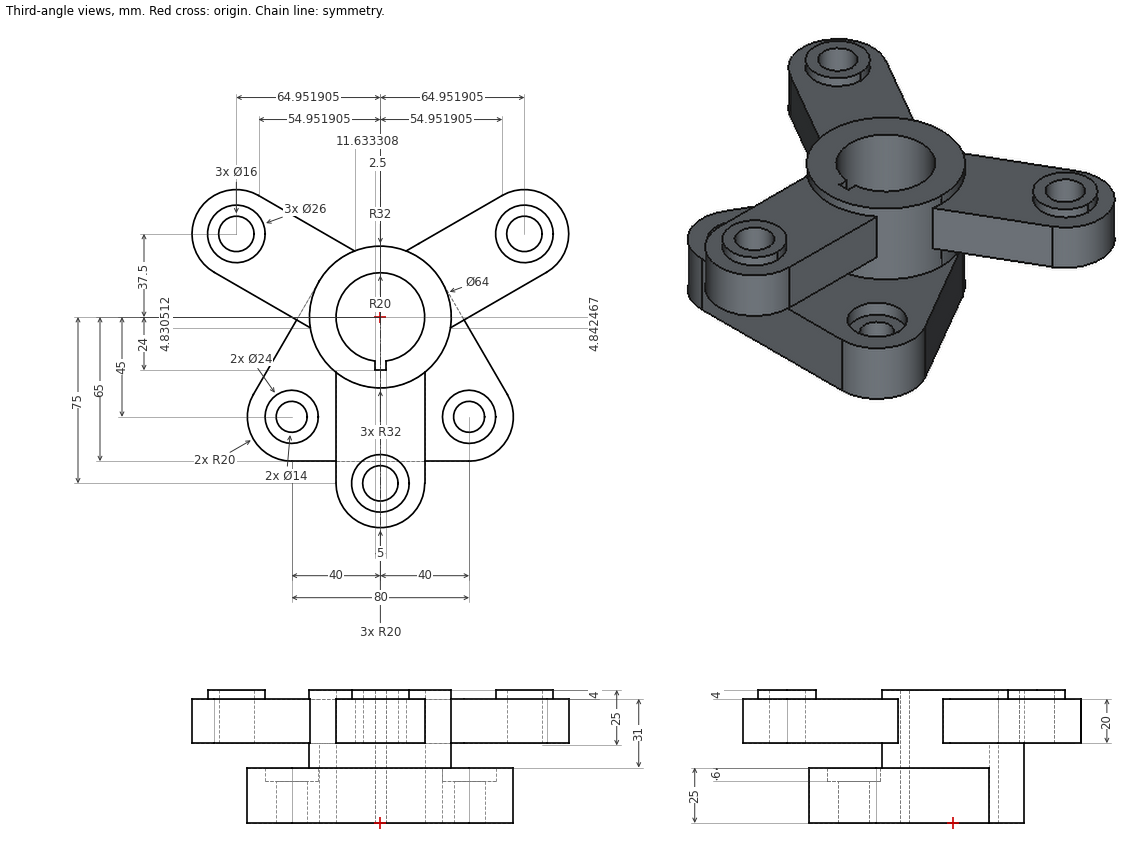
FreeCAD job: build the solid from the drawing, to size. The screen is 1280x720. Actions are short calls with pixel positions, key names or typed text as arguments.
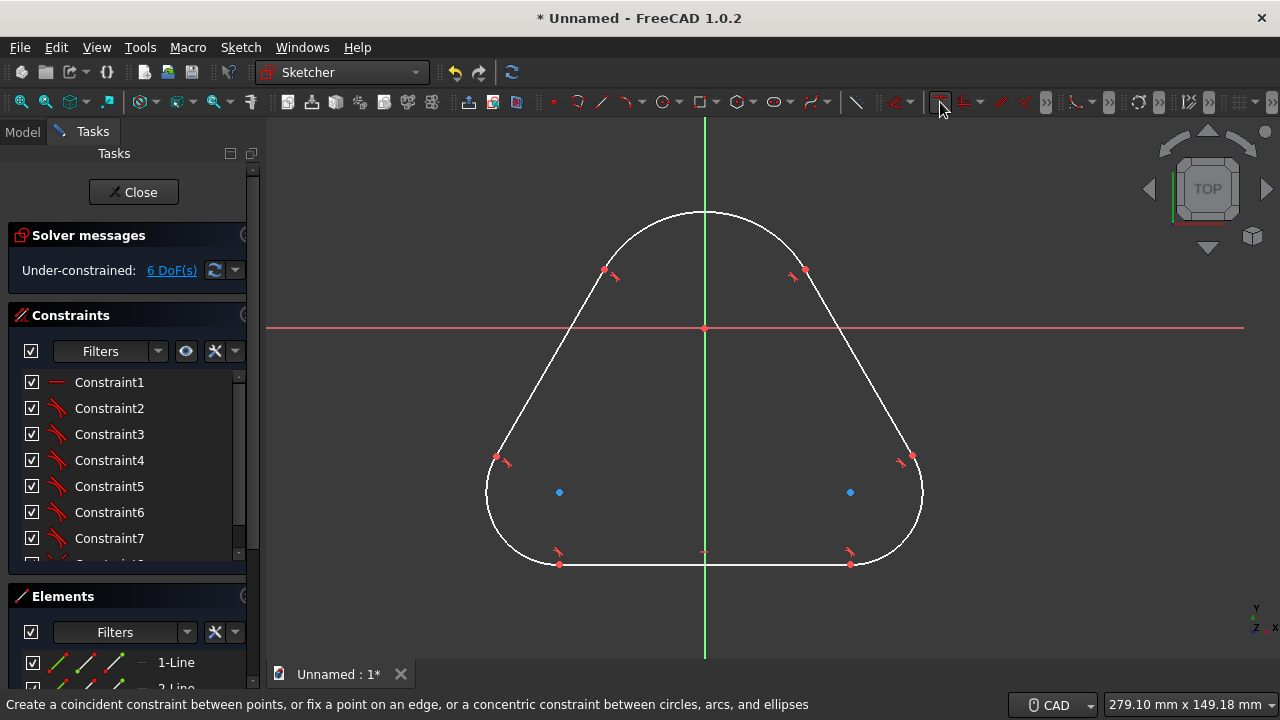
click(487, 500)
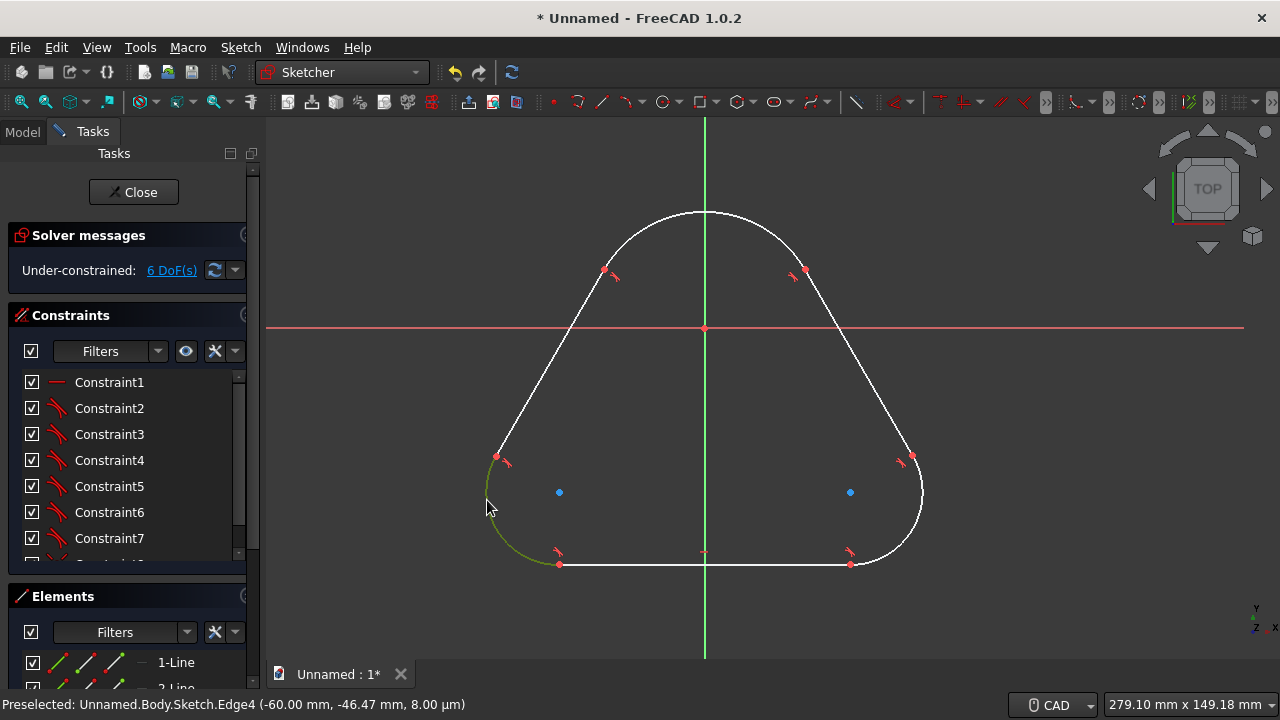
click(893, 551)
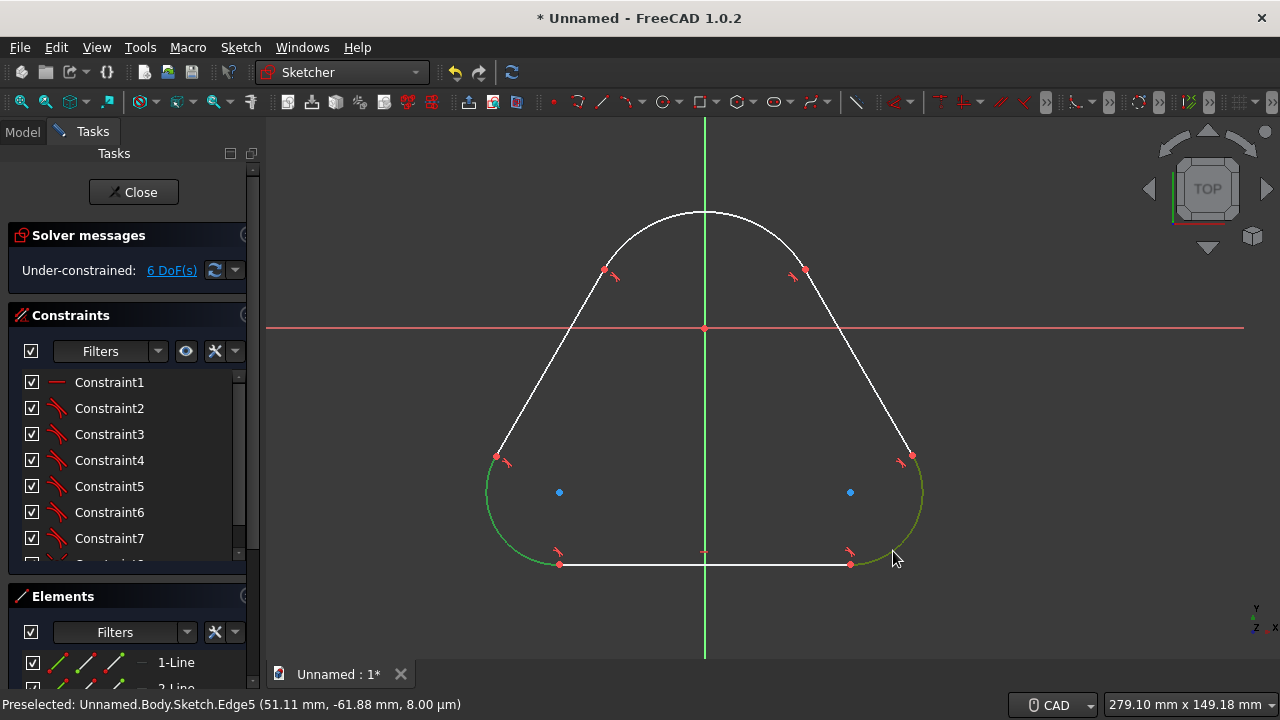
key(e)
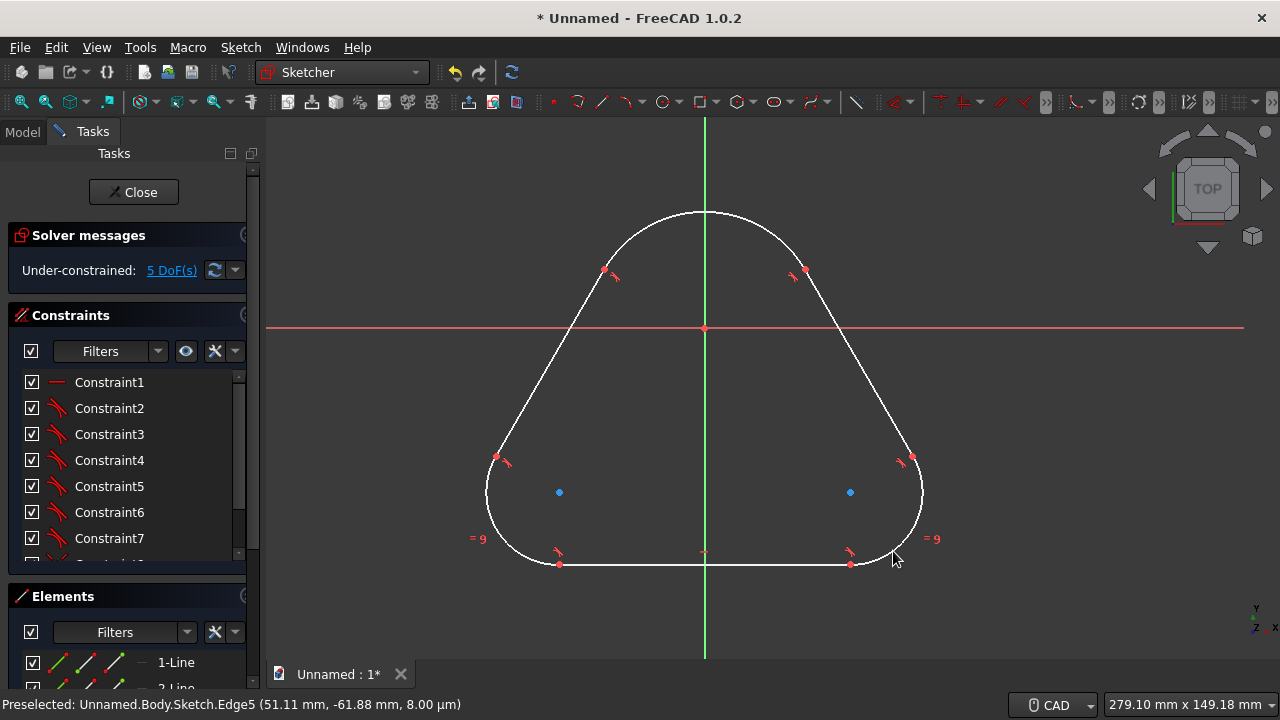
click(487, 500)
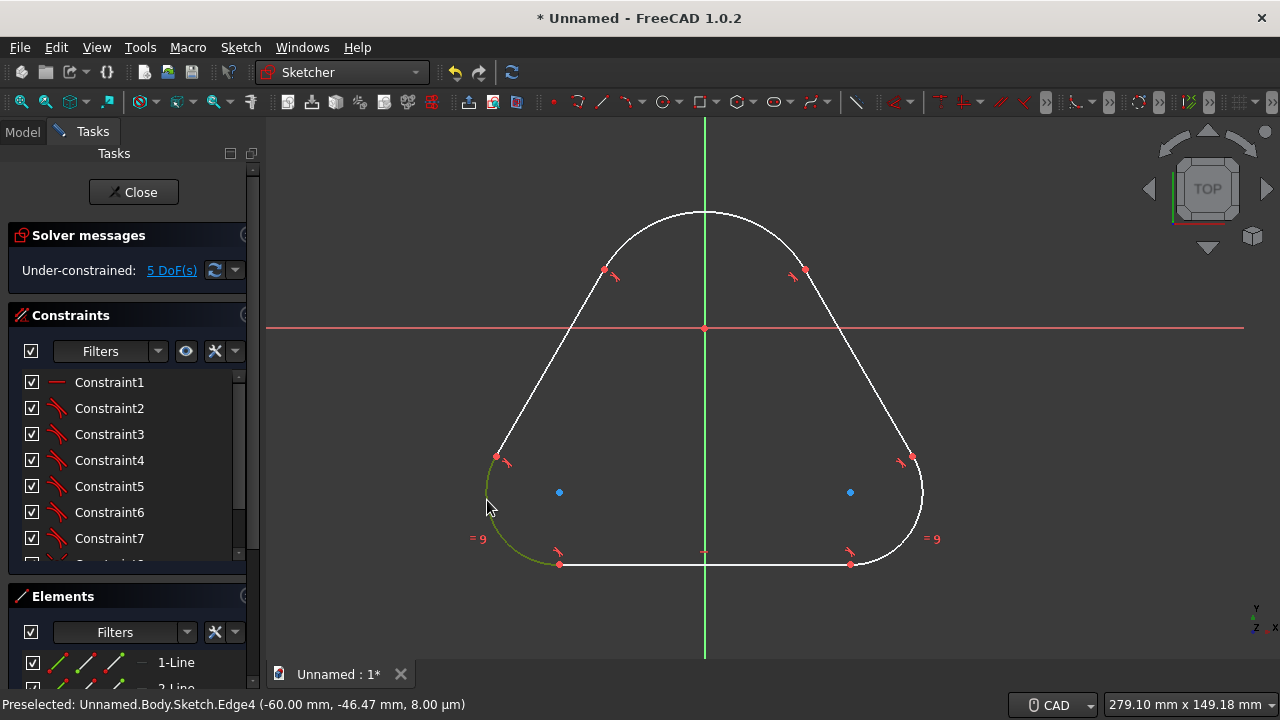
key(k)
key(r)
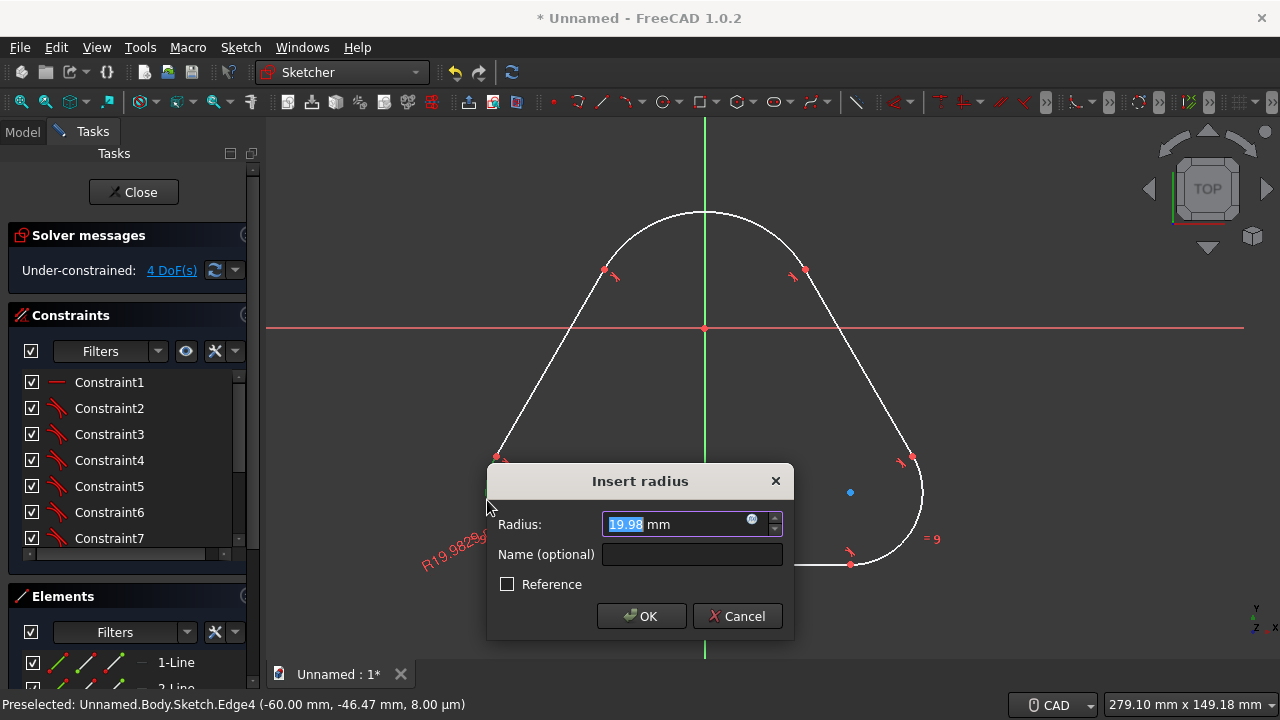
text(20)
key(Return)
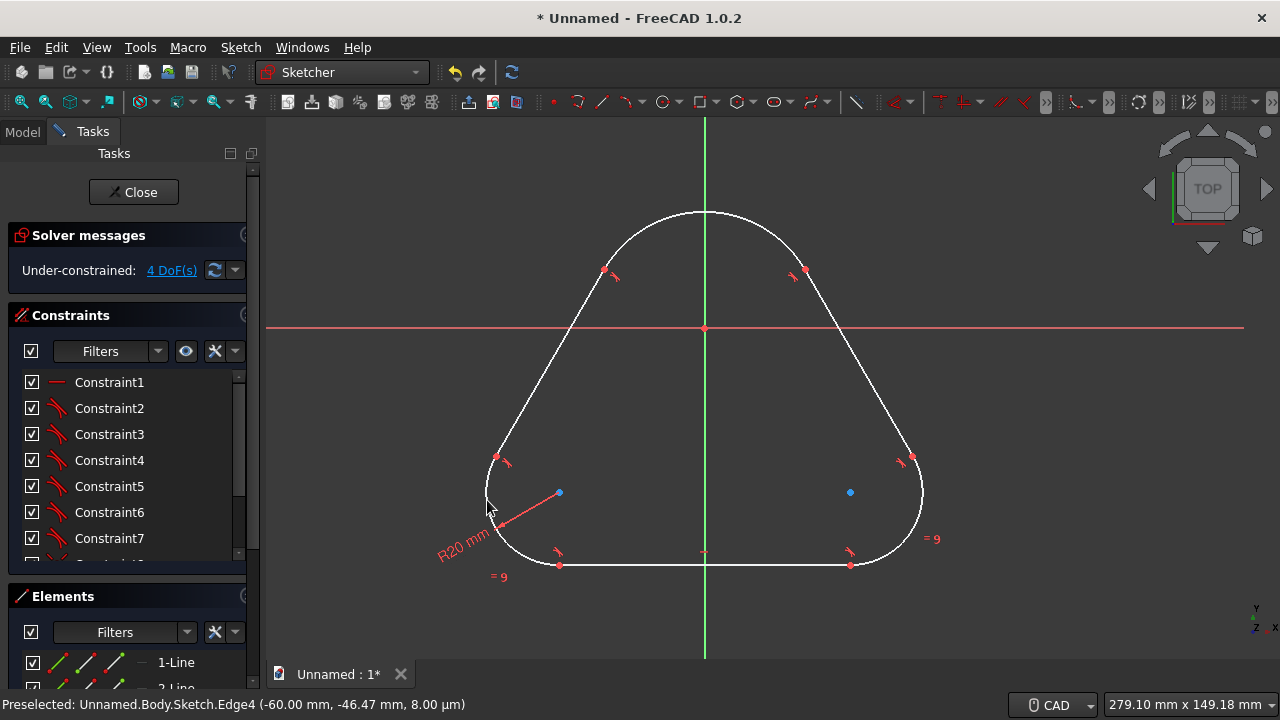
click(752, 222)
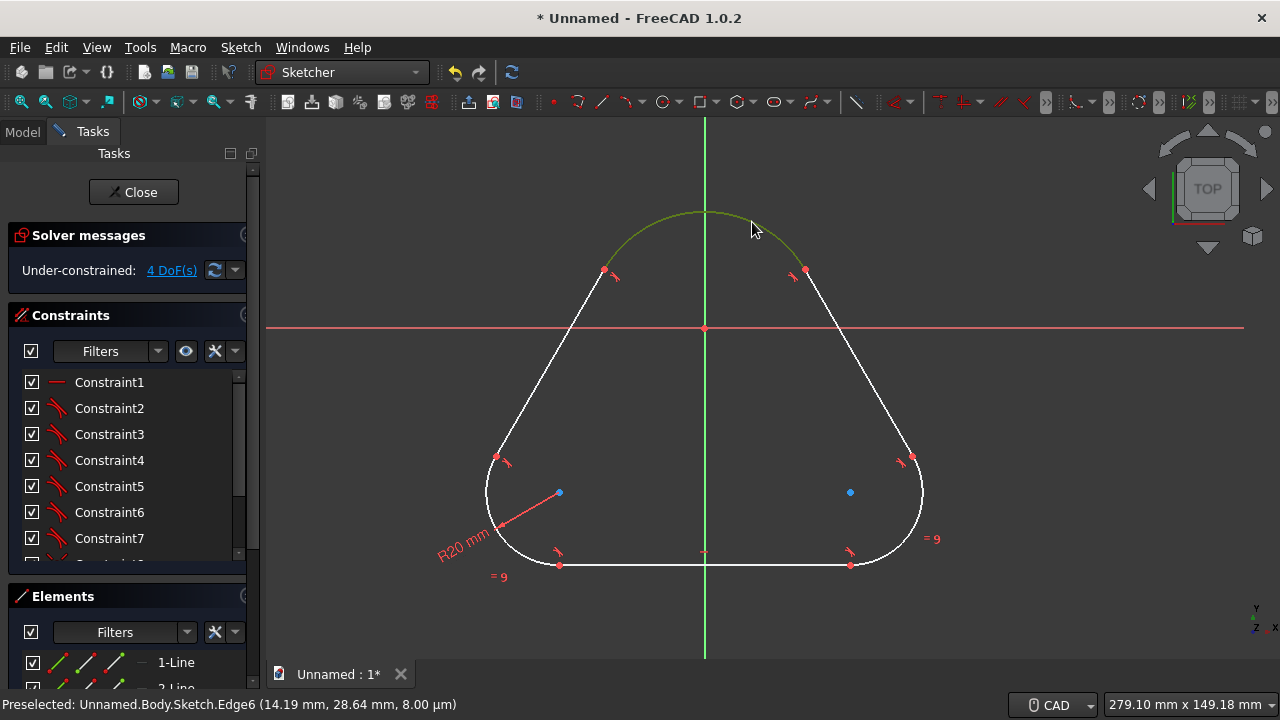
key(k)
key(r)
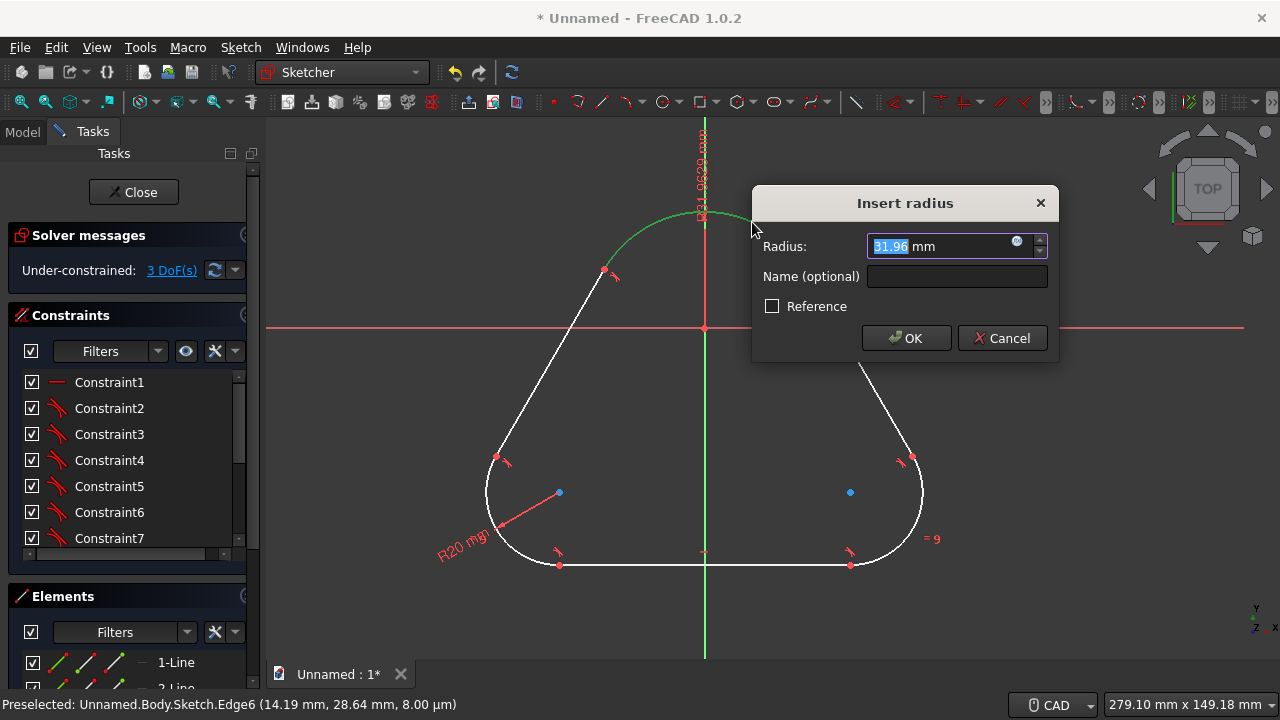
text(32)
key(Return)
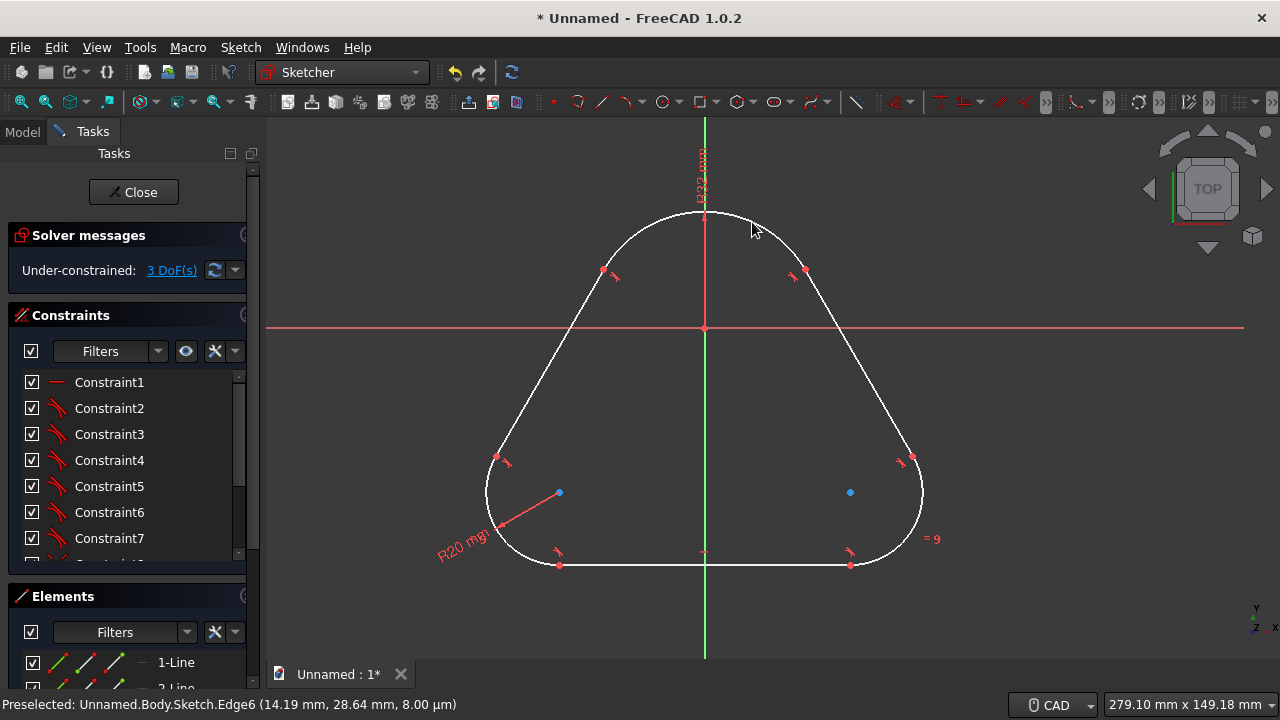
click(646, 565)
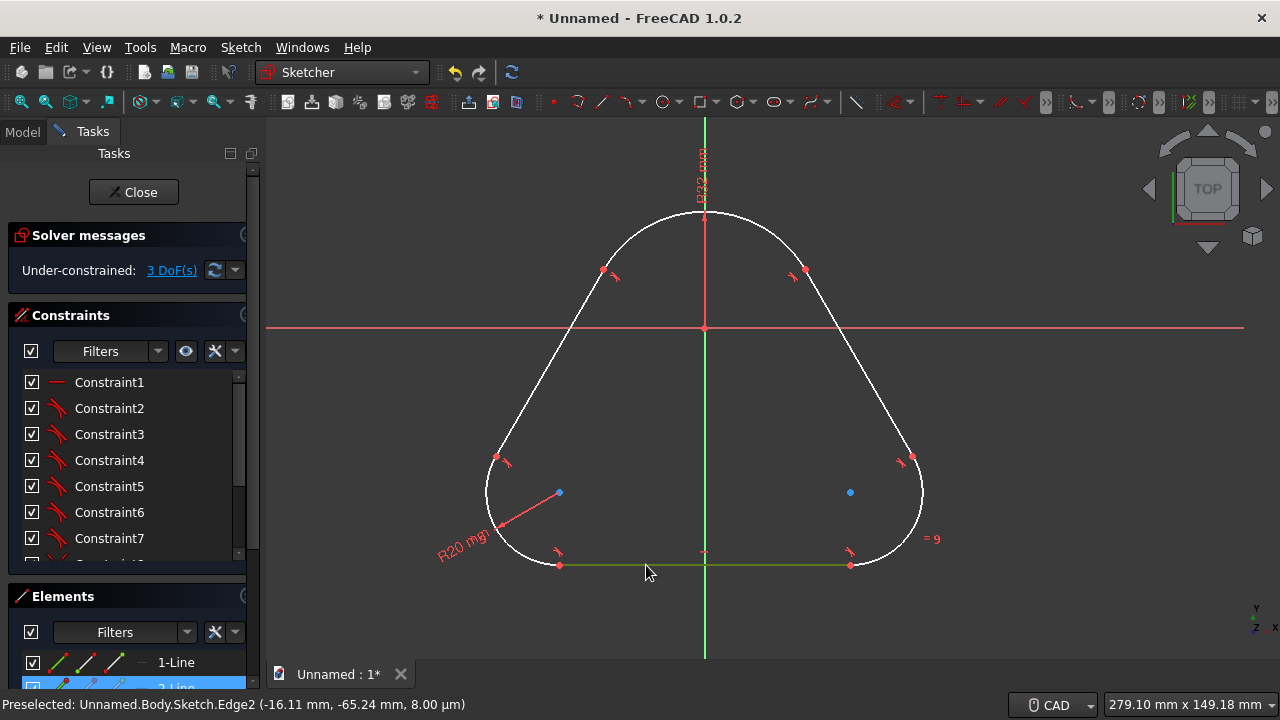
key(l)